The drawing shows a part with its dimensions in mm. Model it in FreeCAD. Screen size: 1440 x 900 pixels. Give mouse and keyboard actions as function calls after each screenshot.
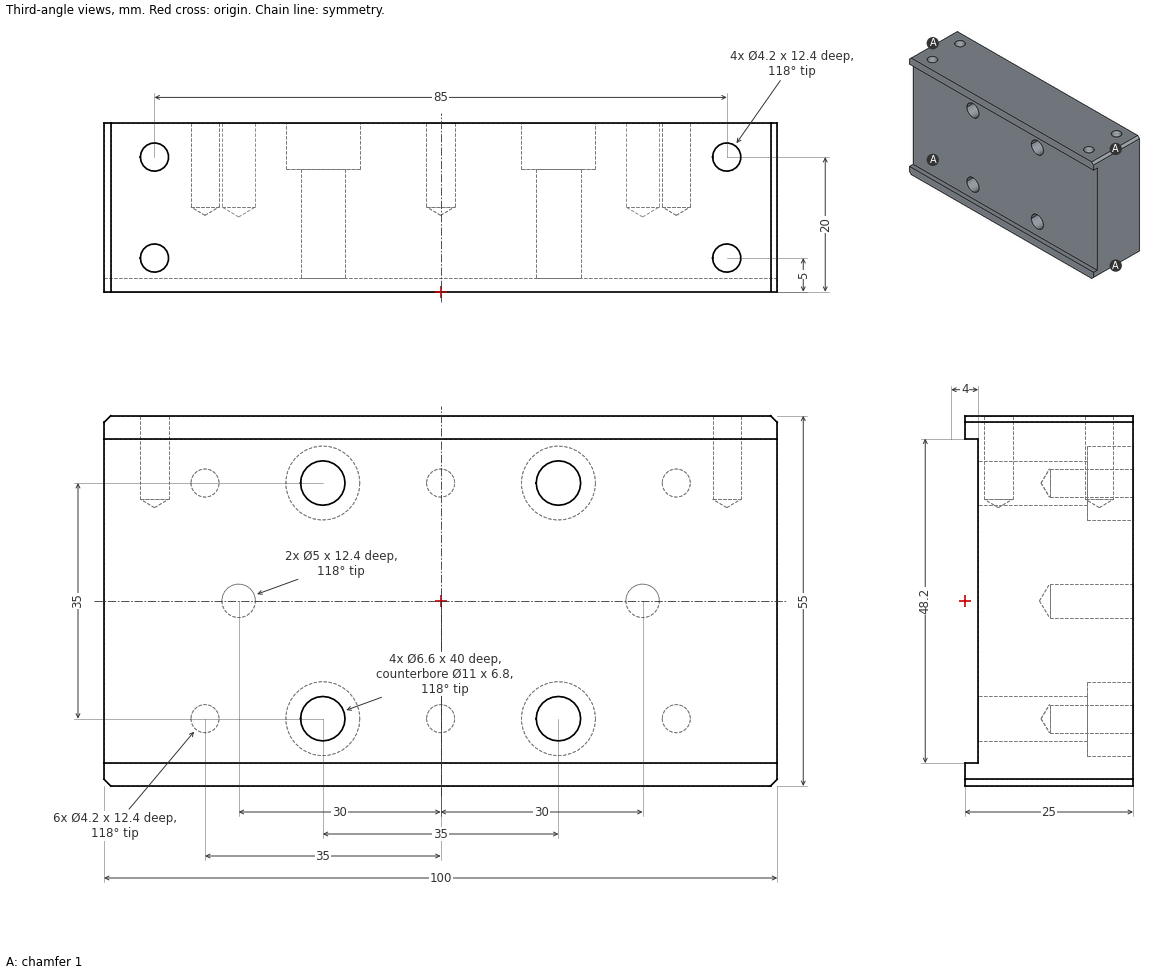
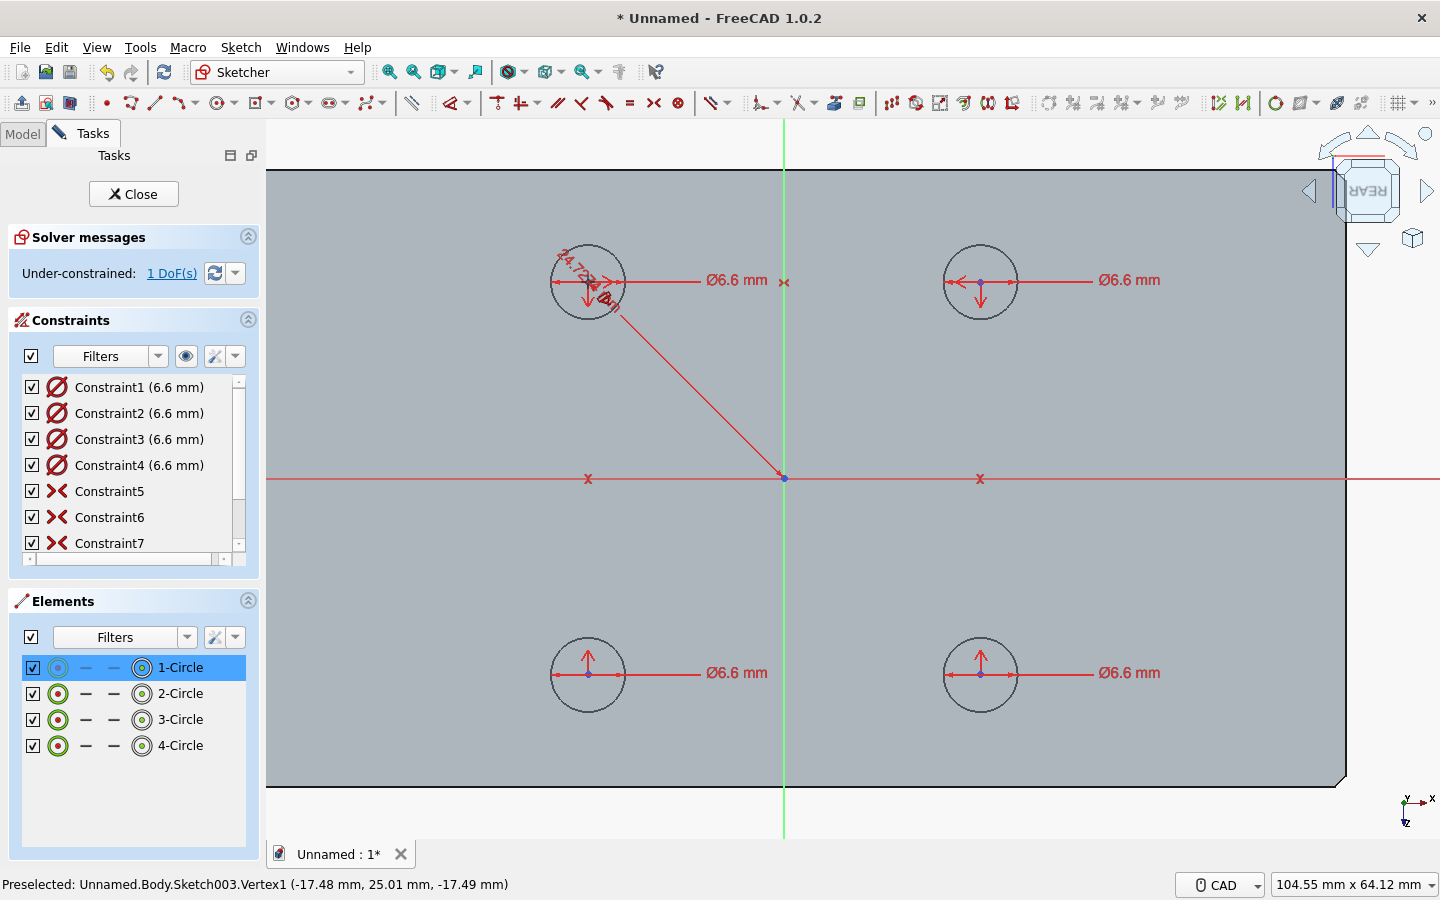
click(981, 282)
click(694, 248)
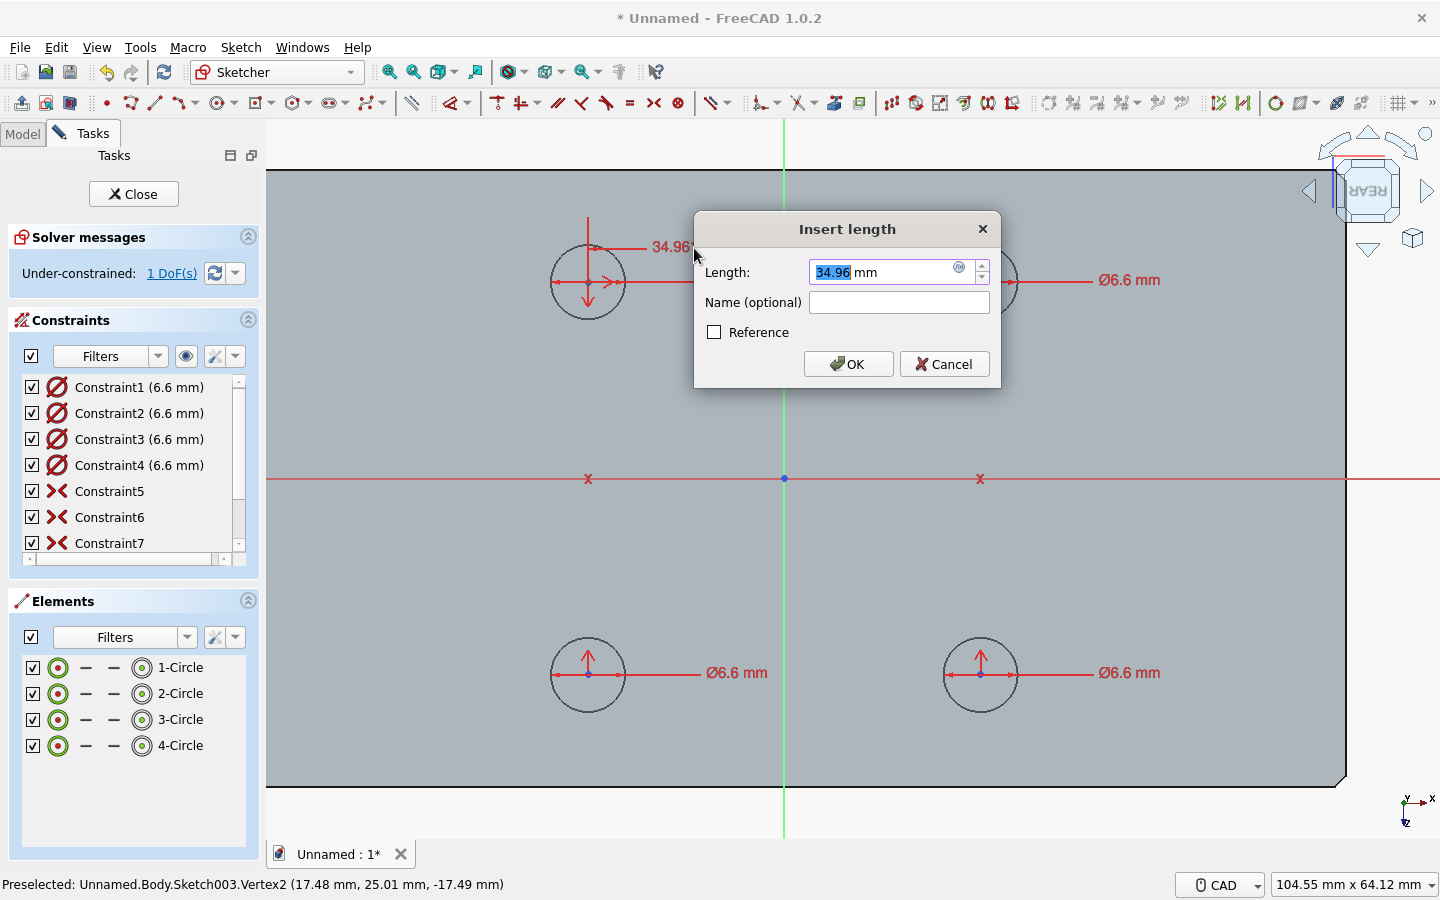
text(35)
key(Return)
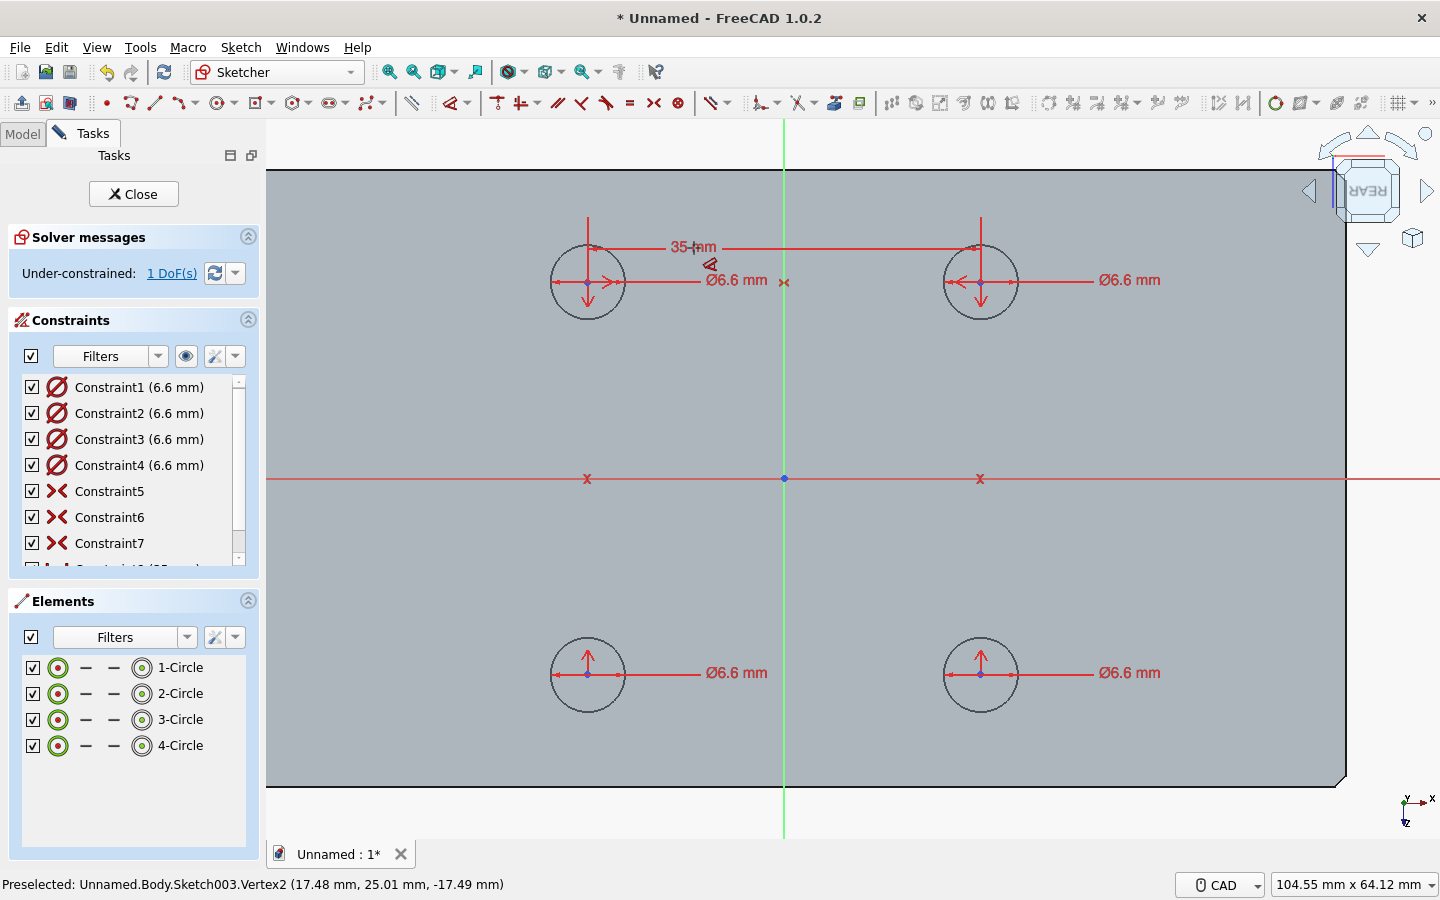
click(588, 282)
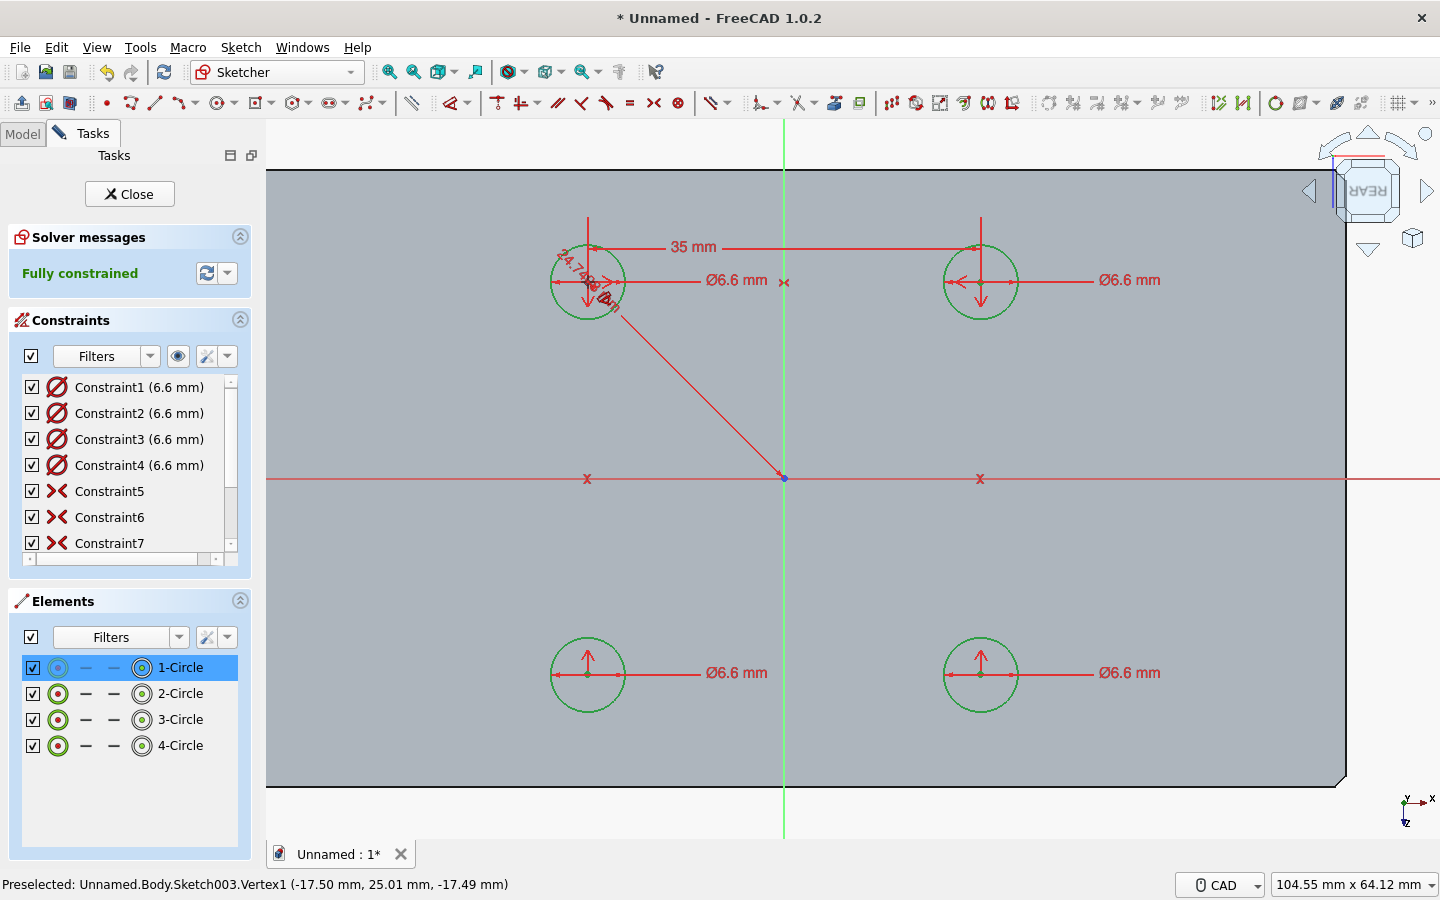
click(588, 675)
click(554, 388)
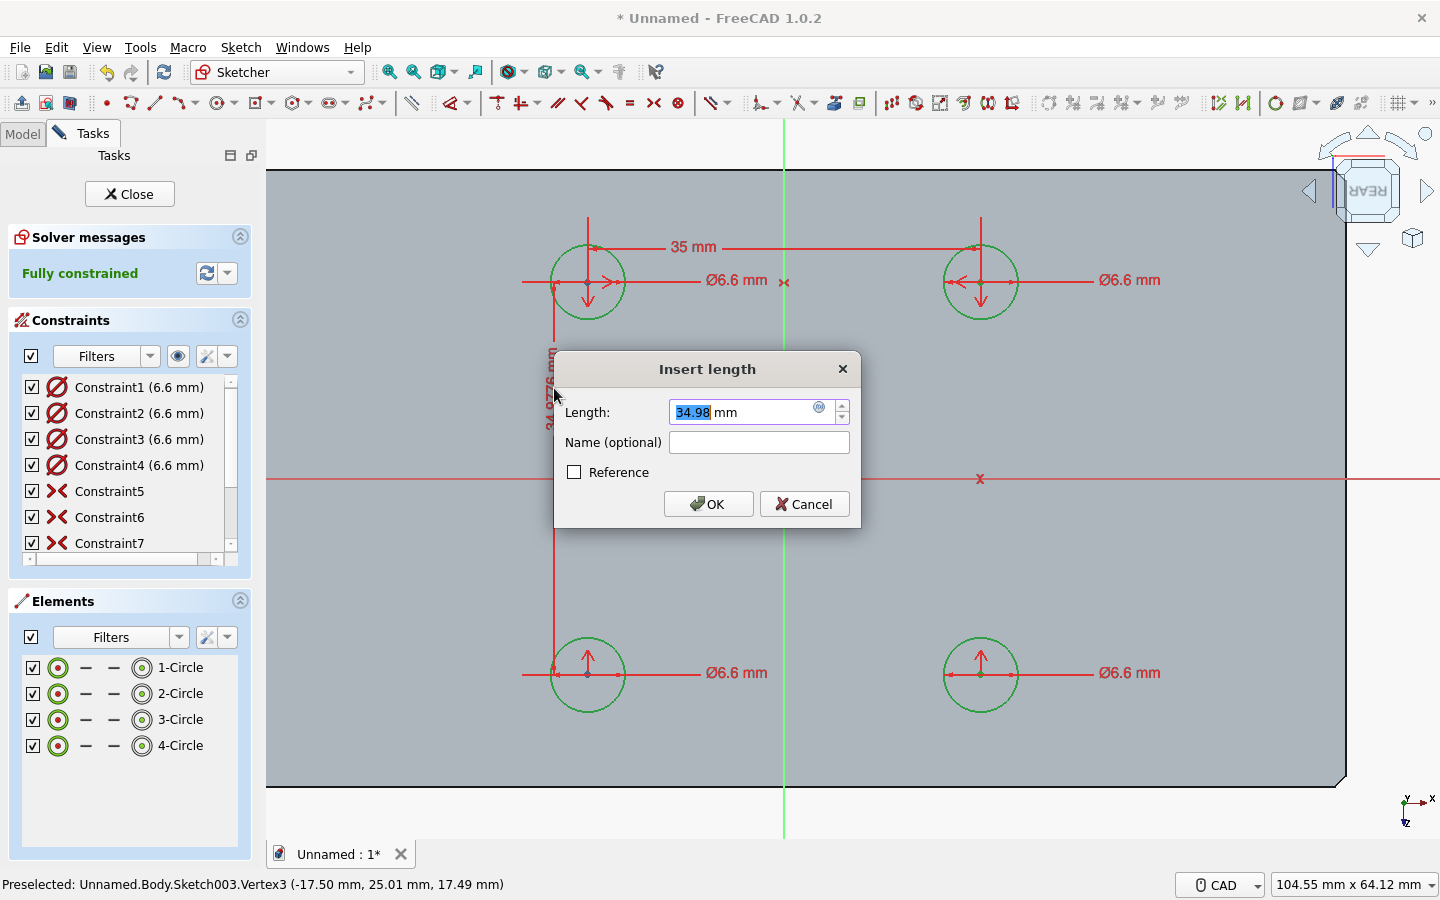
text(35)
key(Return)
key(Escape)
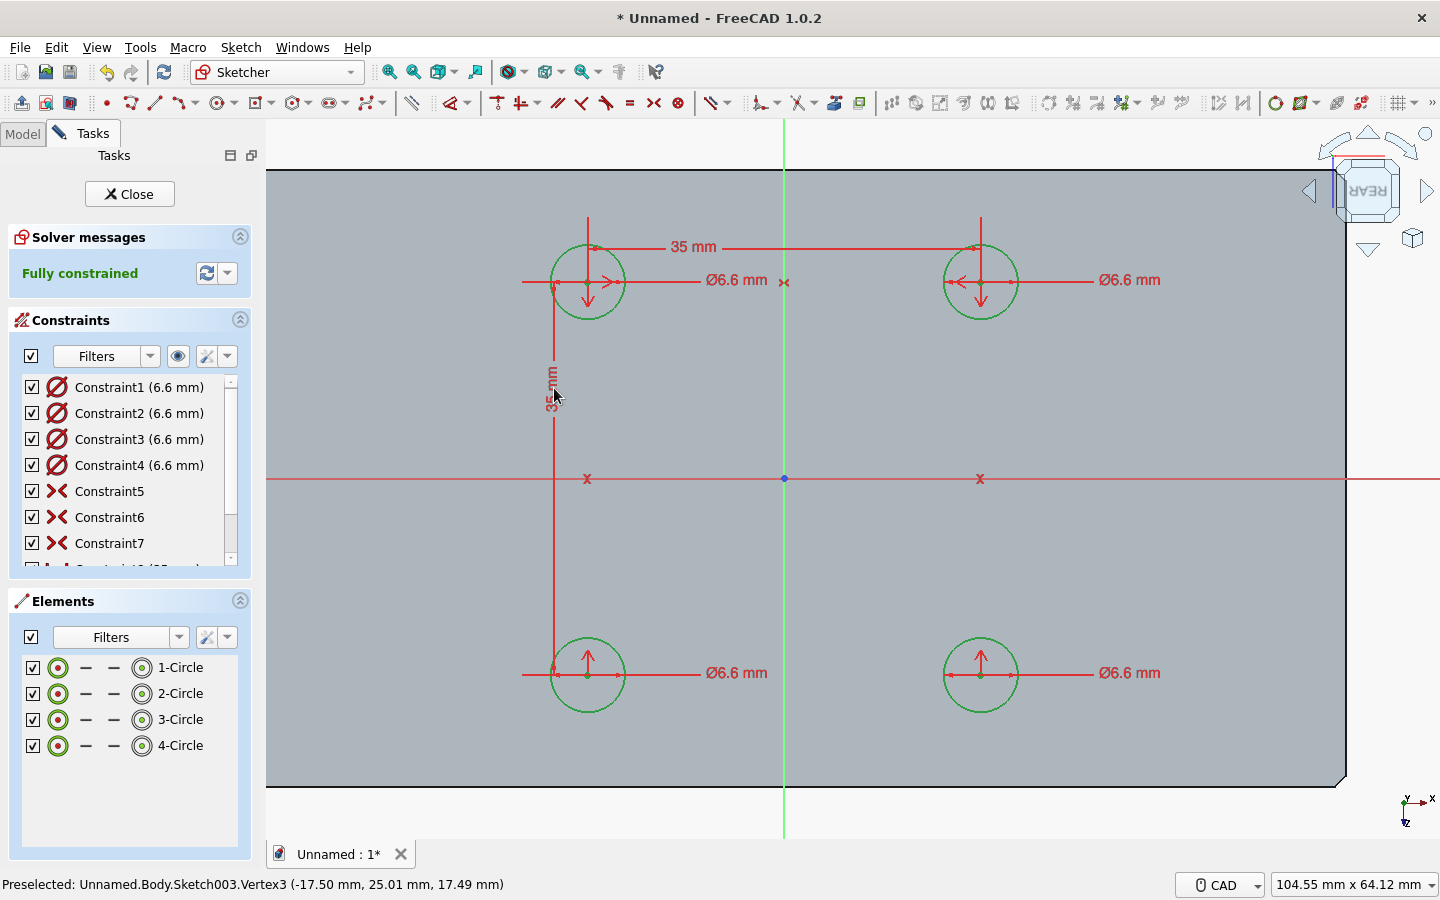
click(130, 194)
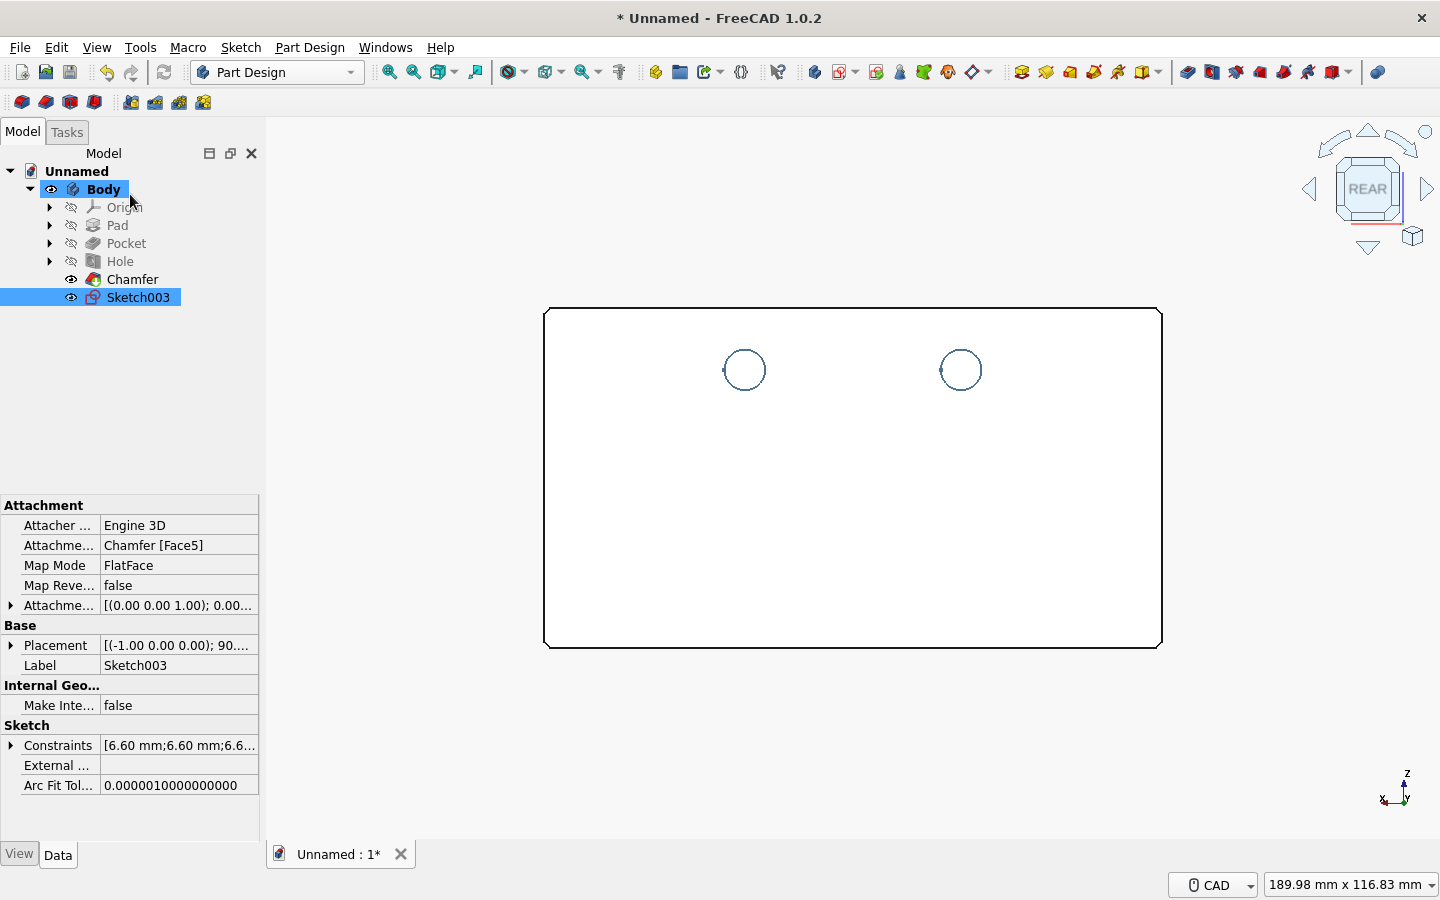
click(1212, 72)